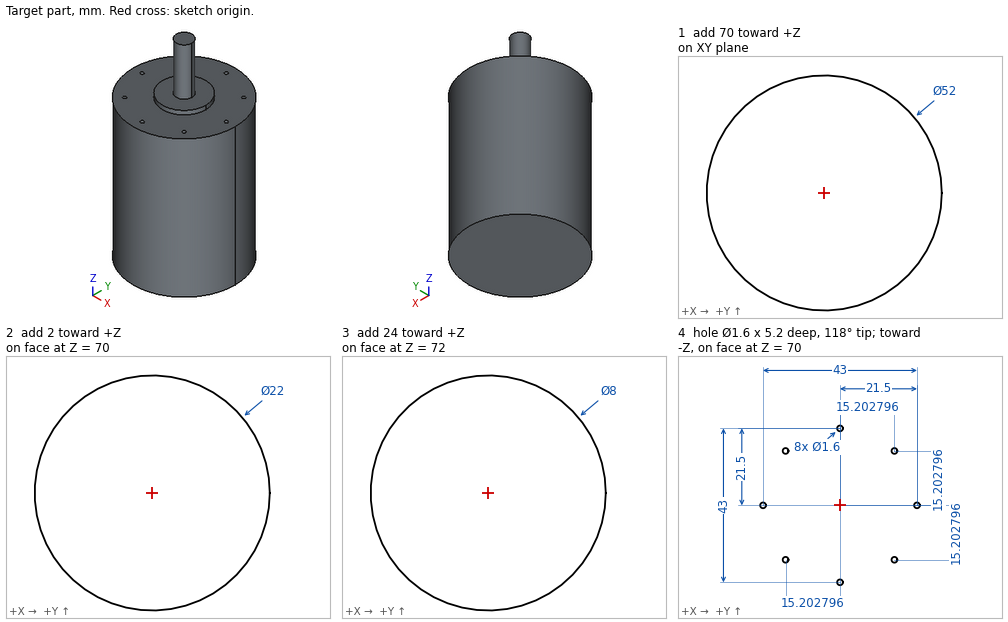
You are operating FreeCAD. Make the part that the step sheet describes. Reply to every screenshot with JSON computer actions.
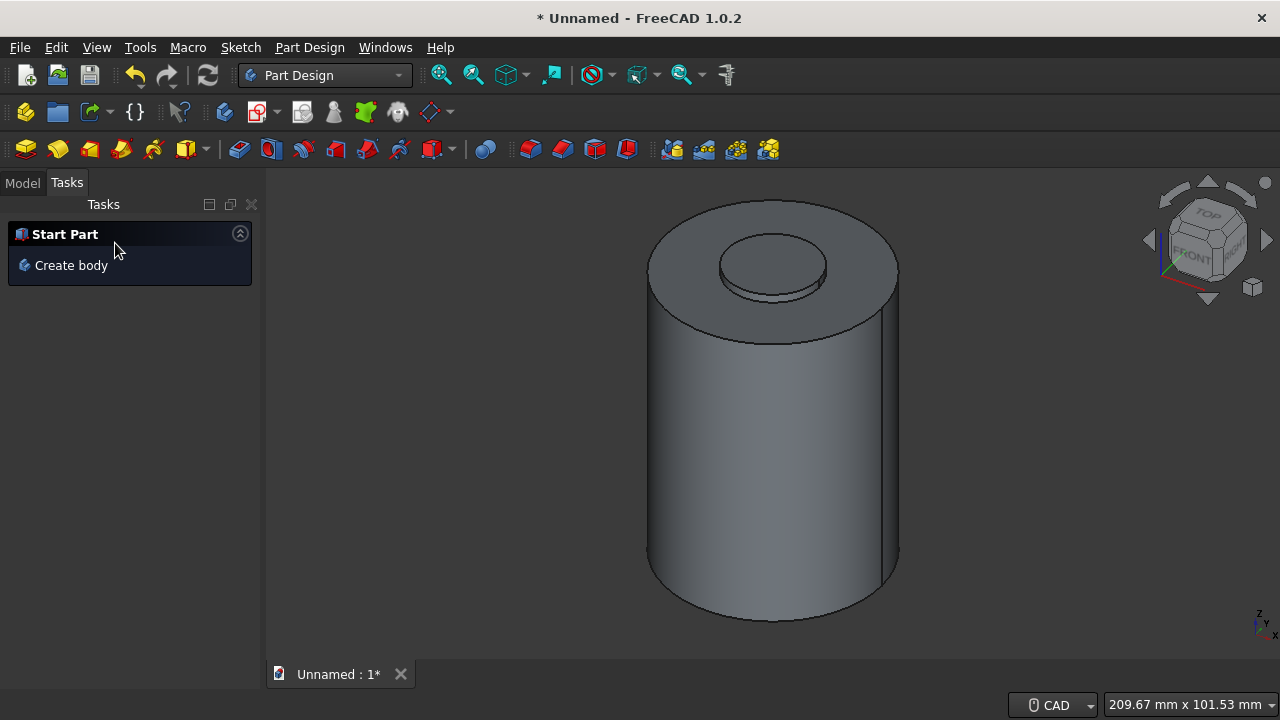
{"action": "left_click", "coordinate": [442, 76]}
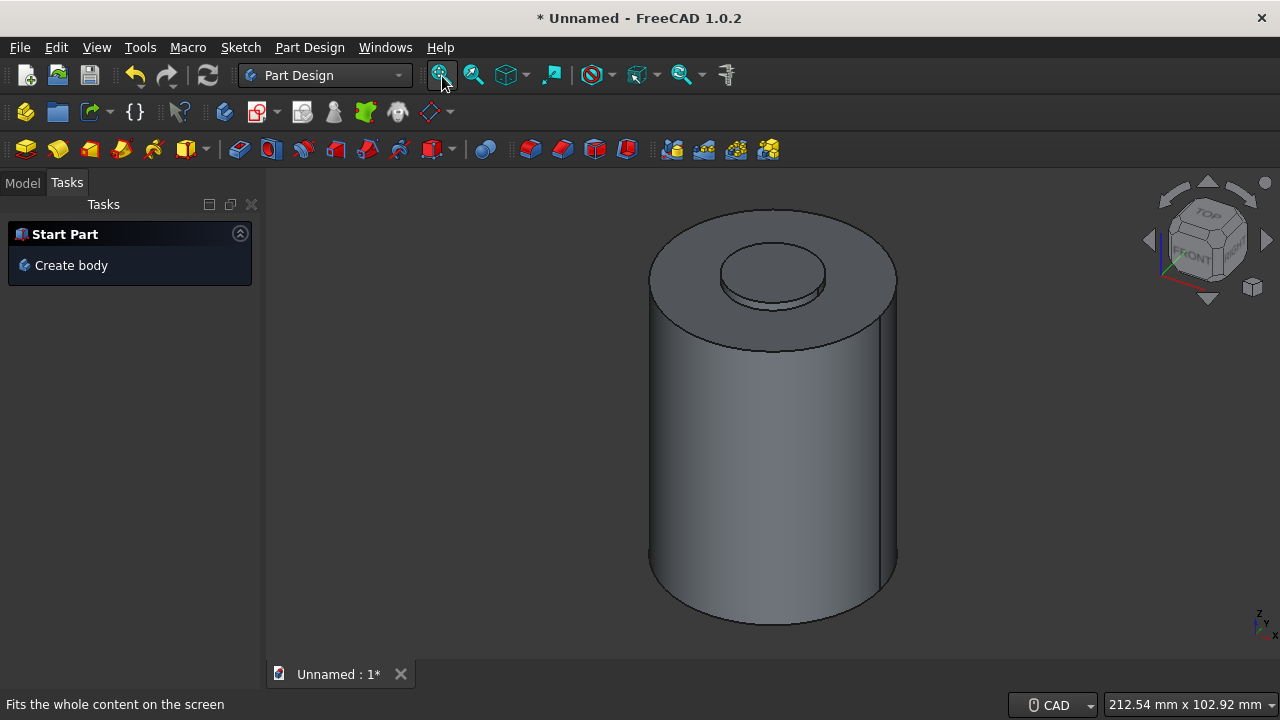
{"action": "left_click", "coordinate": [773, 272]}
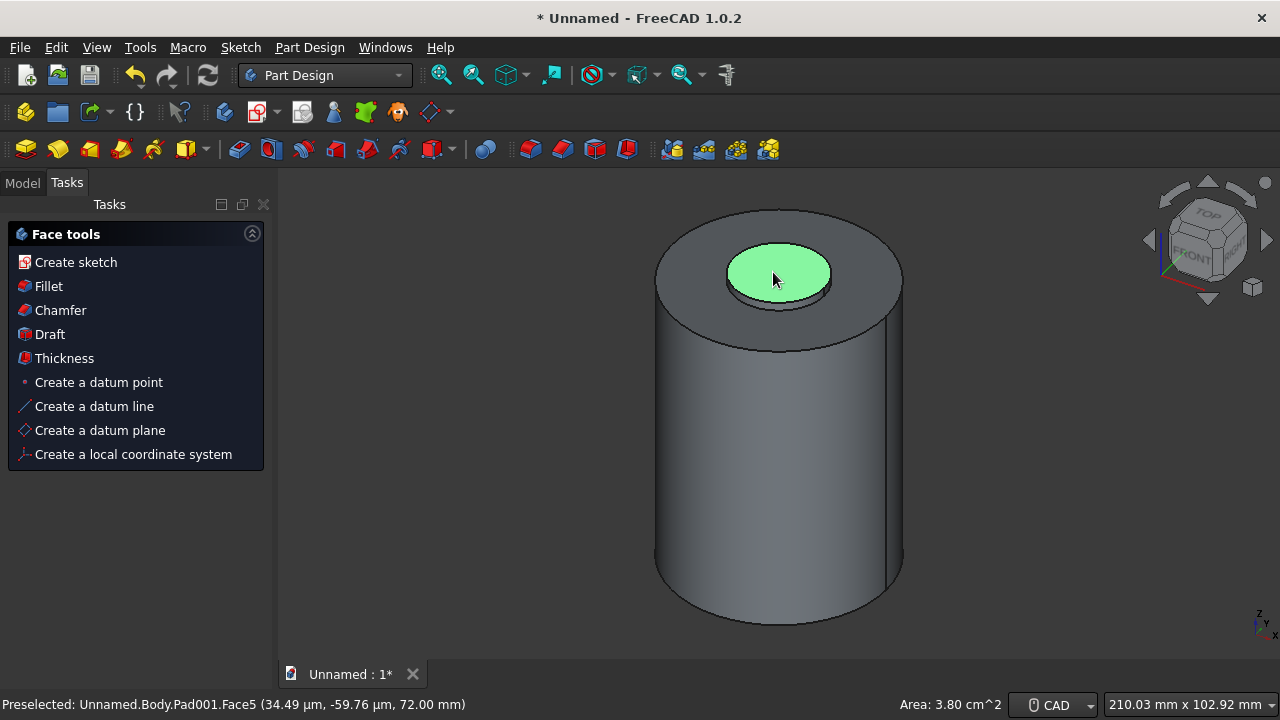
{"action": "left_click", "coordinate": [258, 112]}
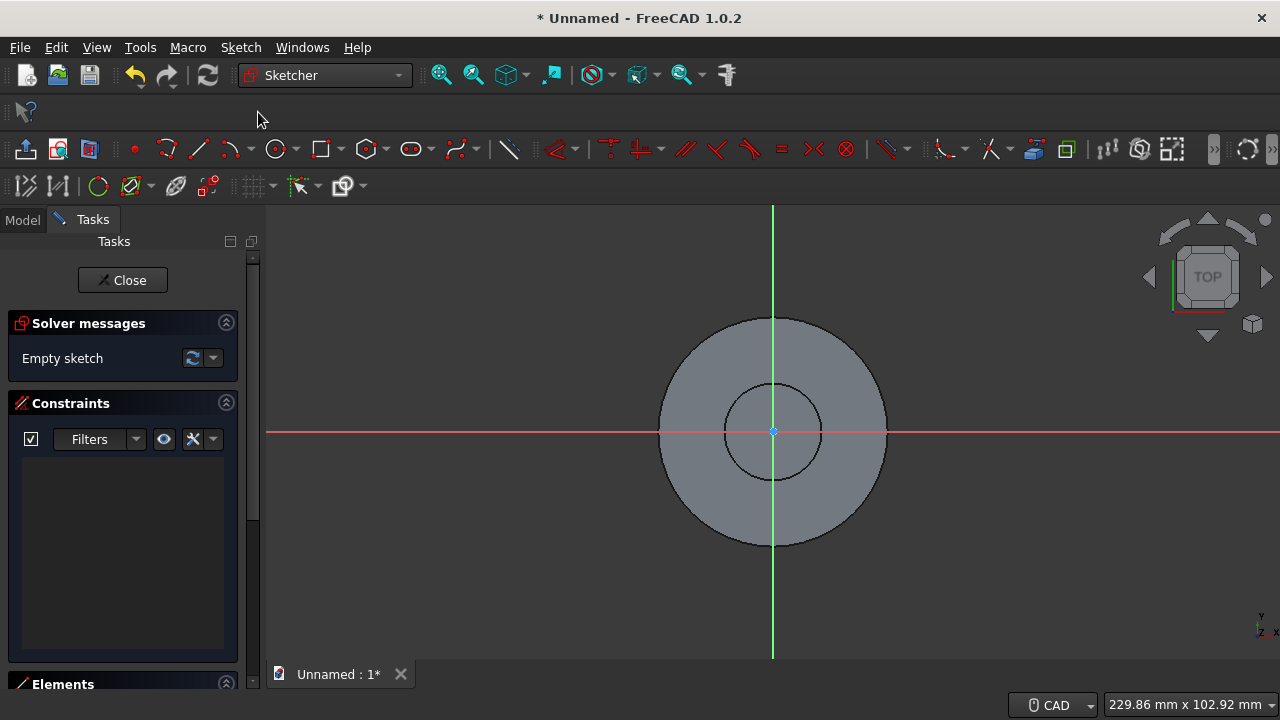
{"action": "scroll", "coordinate": [784, 432], "scroll_direction": "up", "scroll_amount": 10}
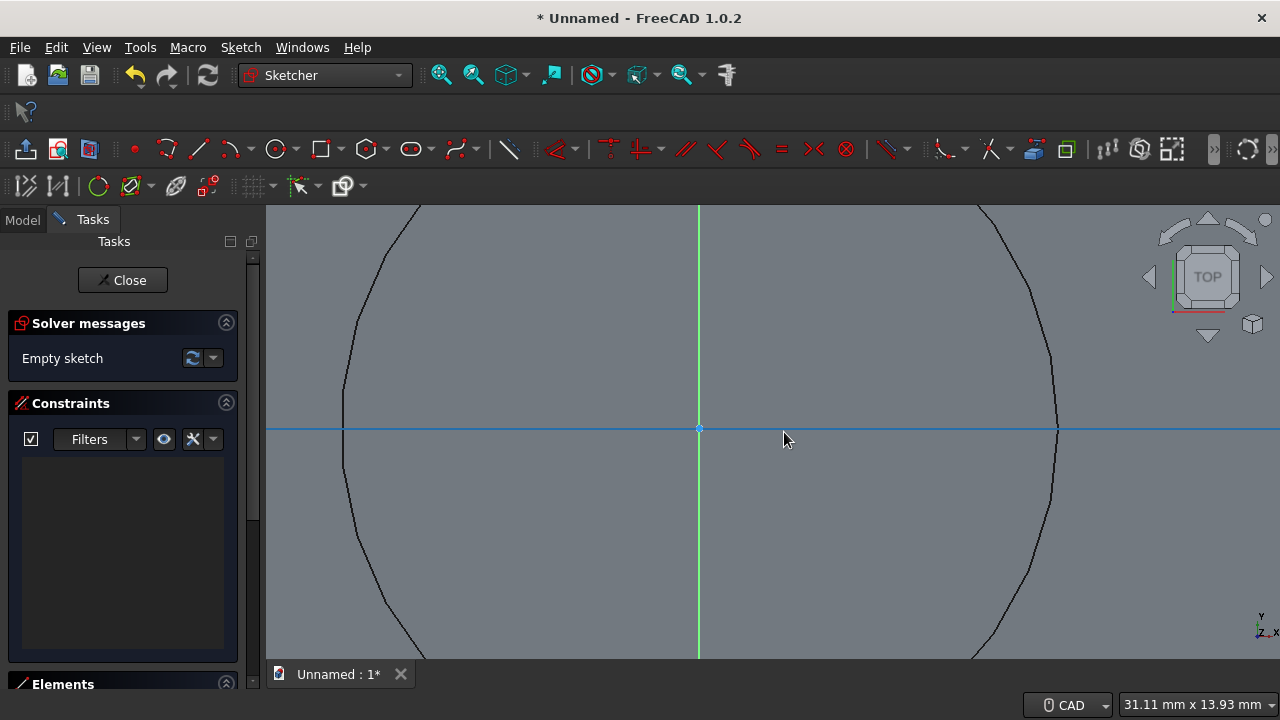
{"action": "left_click", "coordinate": [276, 150]}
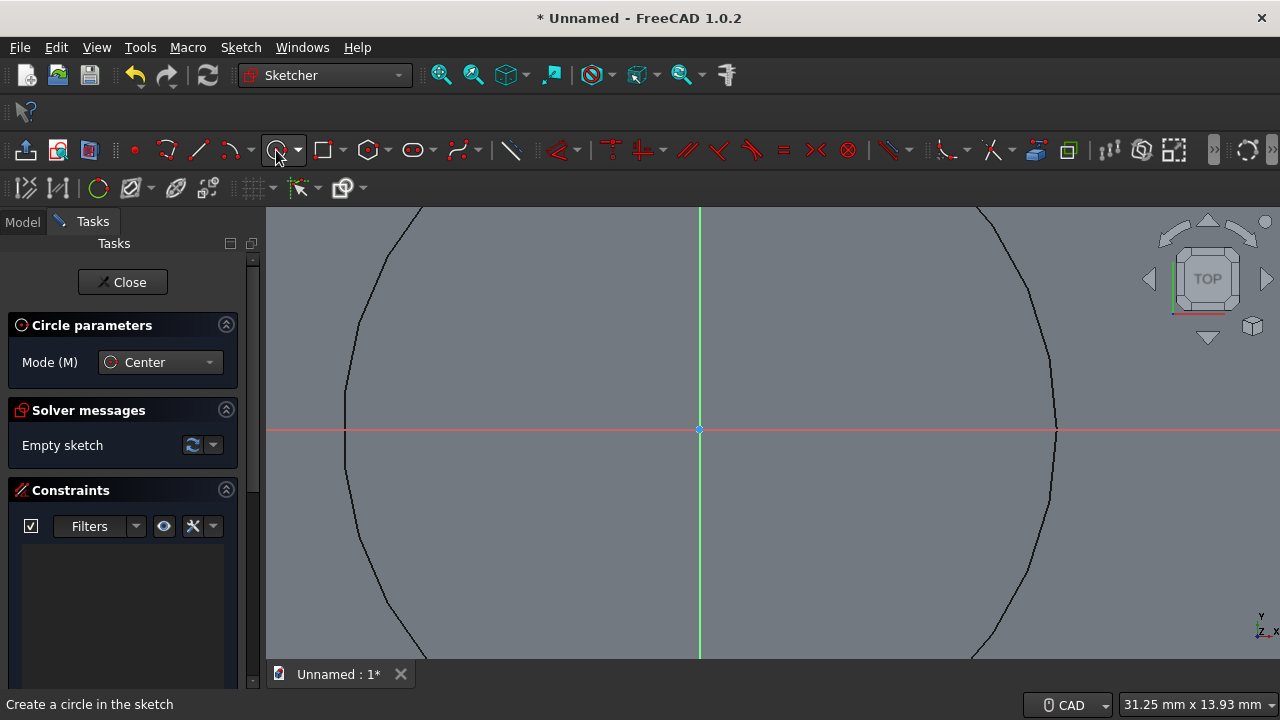
{"action": "left_click", "coordinate": [700, 430]}
{"action": "mouse_move", "coordinate": [792, 338]}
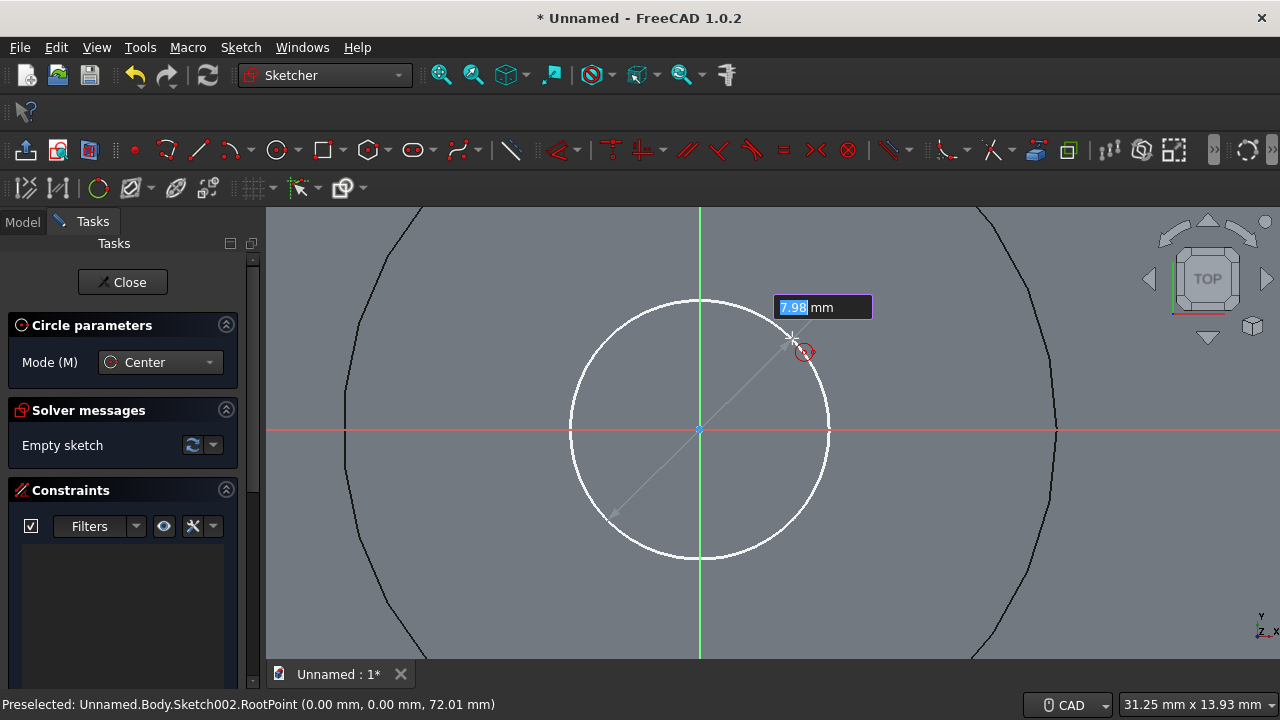
{"action": "type", "text": "8"}
{"action": "key", "text": "Return"}
{"action": "key", "text": "Escape"}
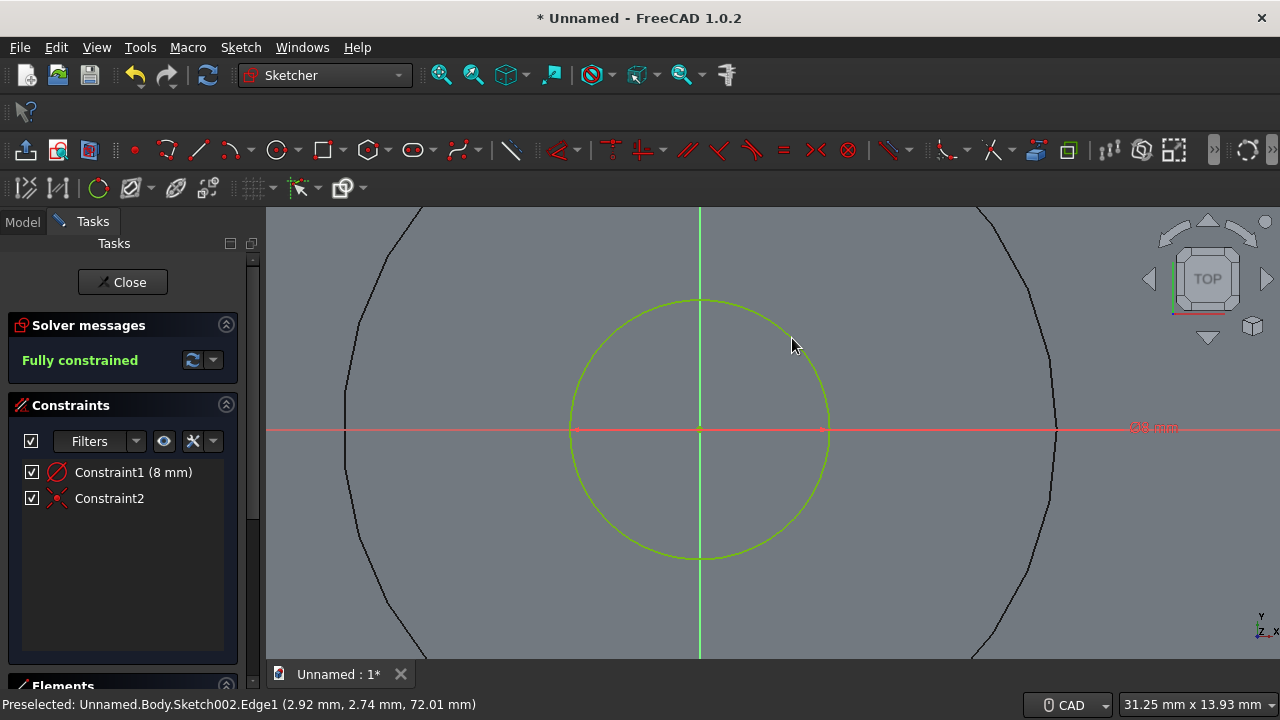
{"action": "left_click", "coordinate": [123, 282]}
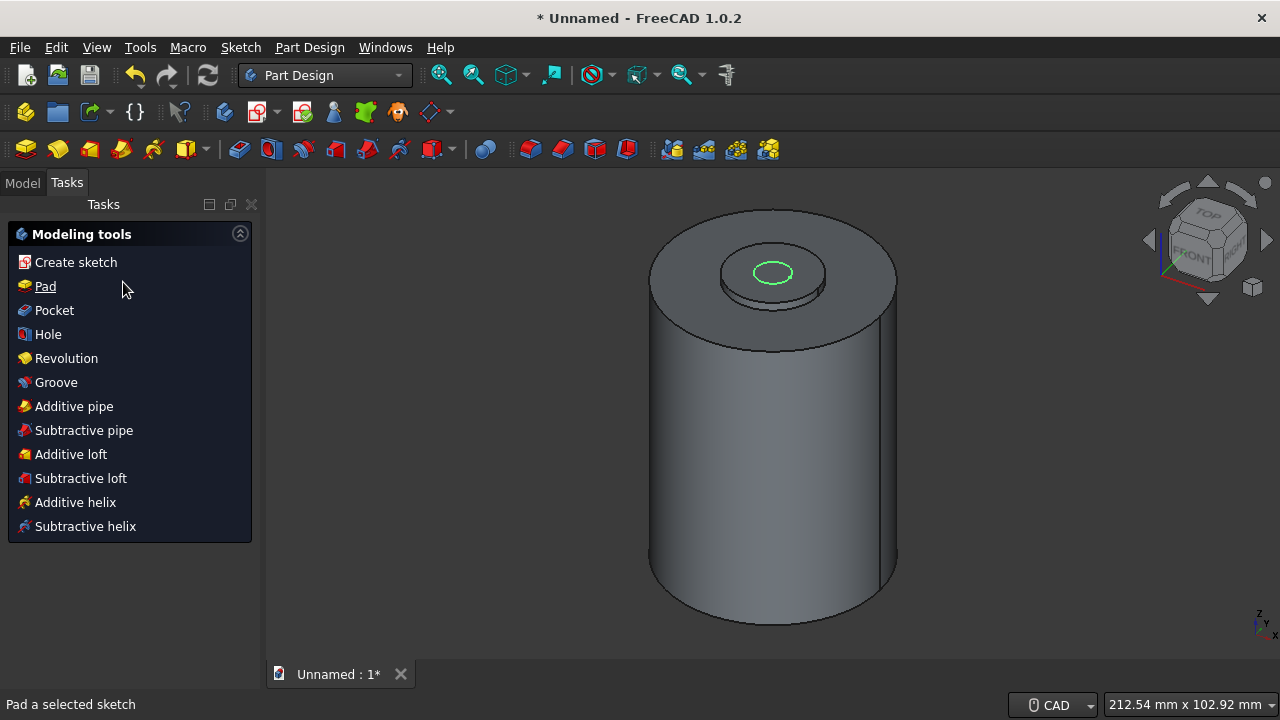
{"action": "left_click", "coordinate": [26, 150]}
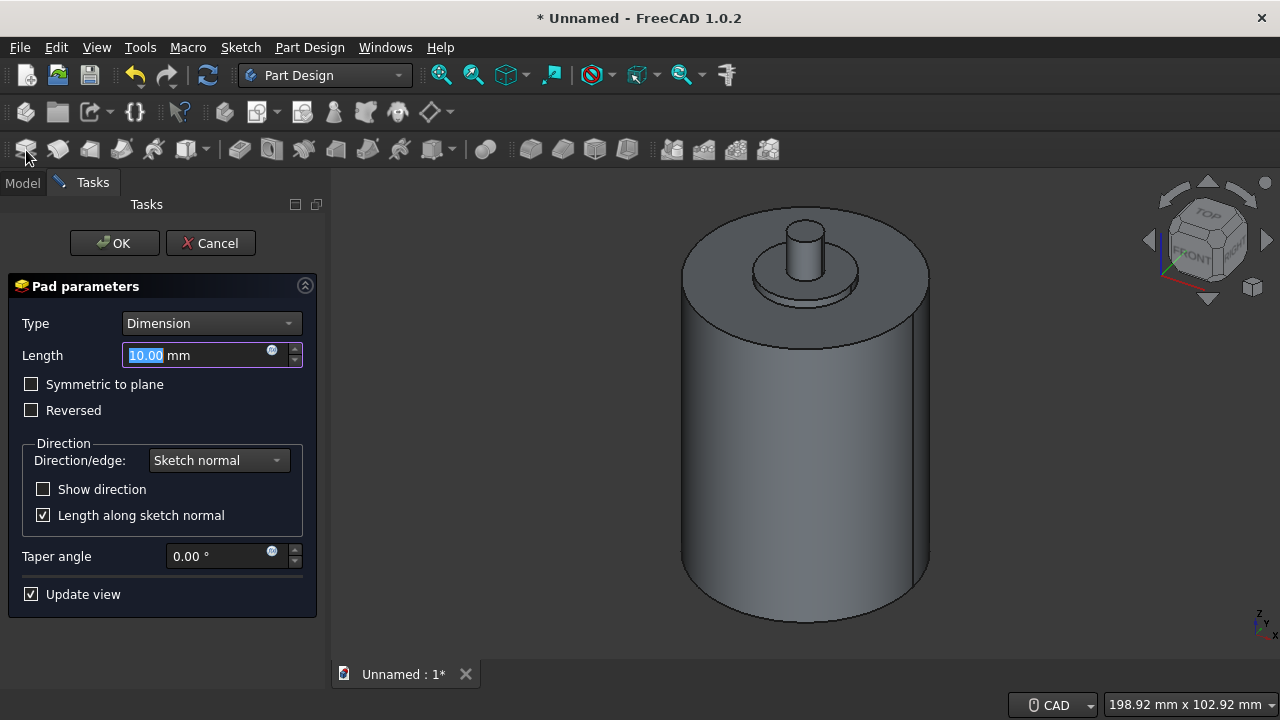
{"action": "type", "text": "24"}
{"action": "key", "text": "Tab"}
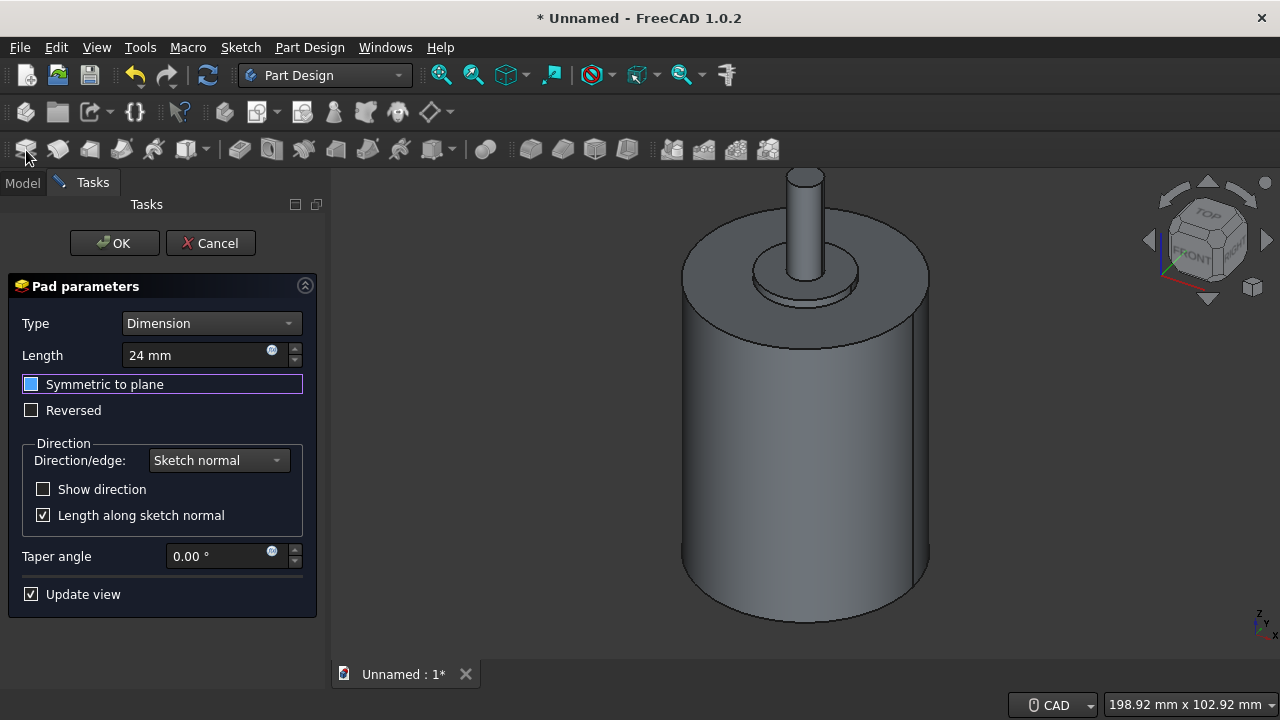
{"action": "left_click", "coordinate": [115, 243]}